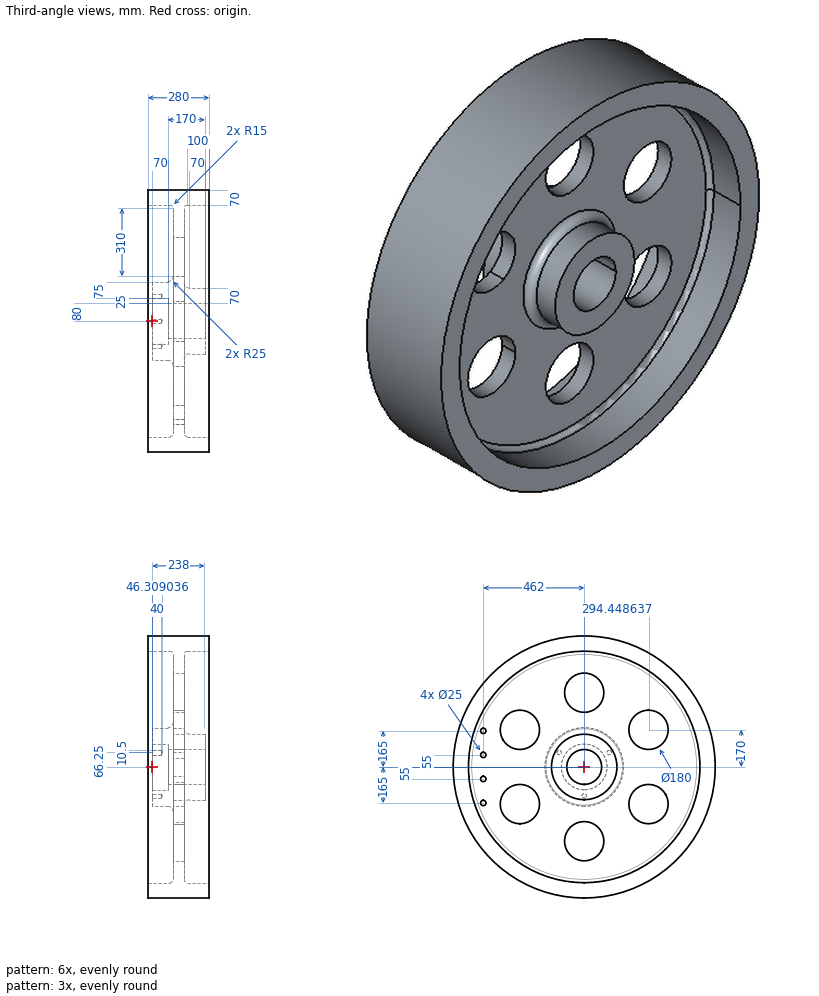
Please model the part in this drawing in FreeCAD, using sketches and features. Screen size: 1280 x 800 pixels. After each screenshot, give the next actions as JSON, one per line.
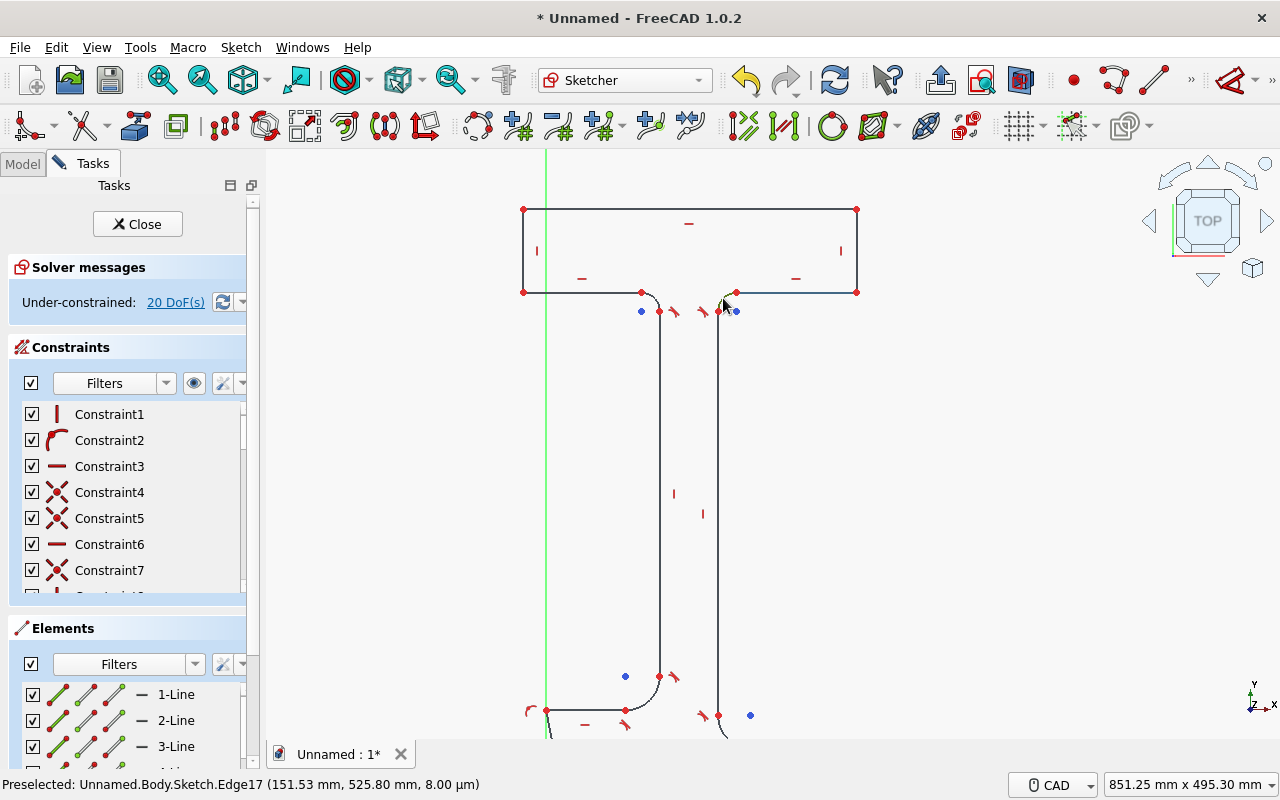
{"action": "key", "text": "t"}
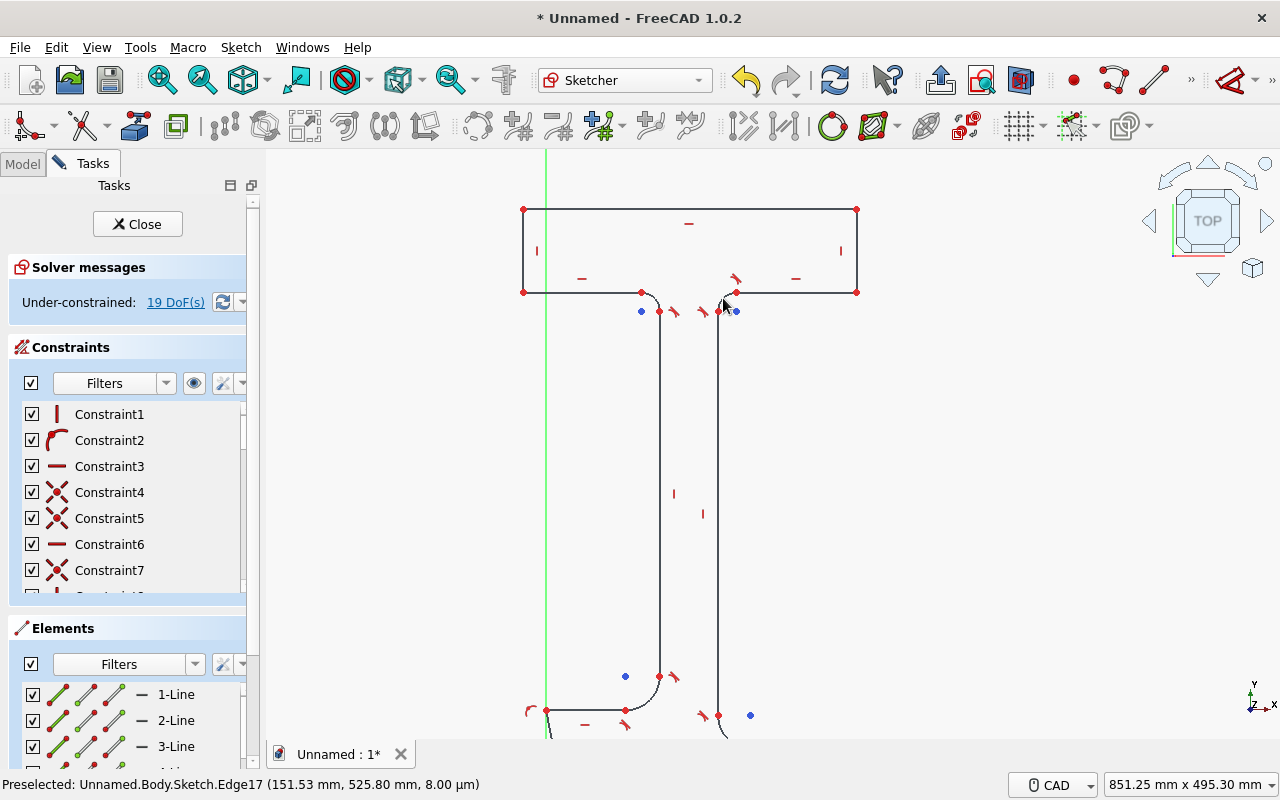
{"action": "left_click", "coordinate": [559, 293]}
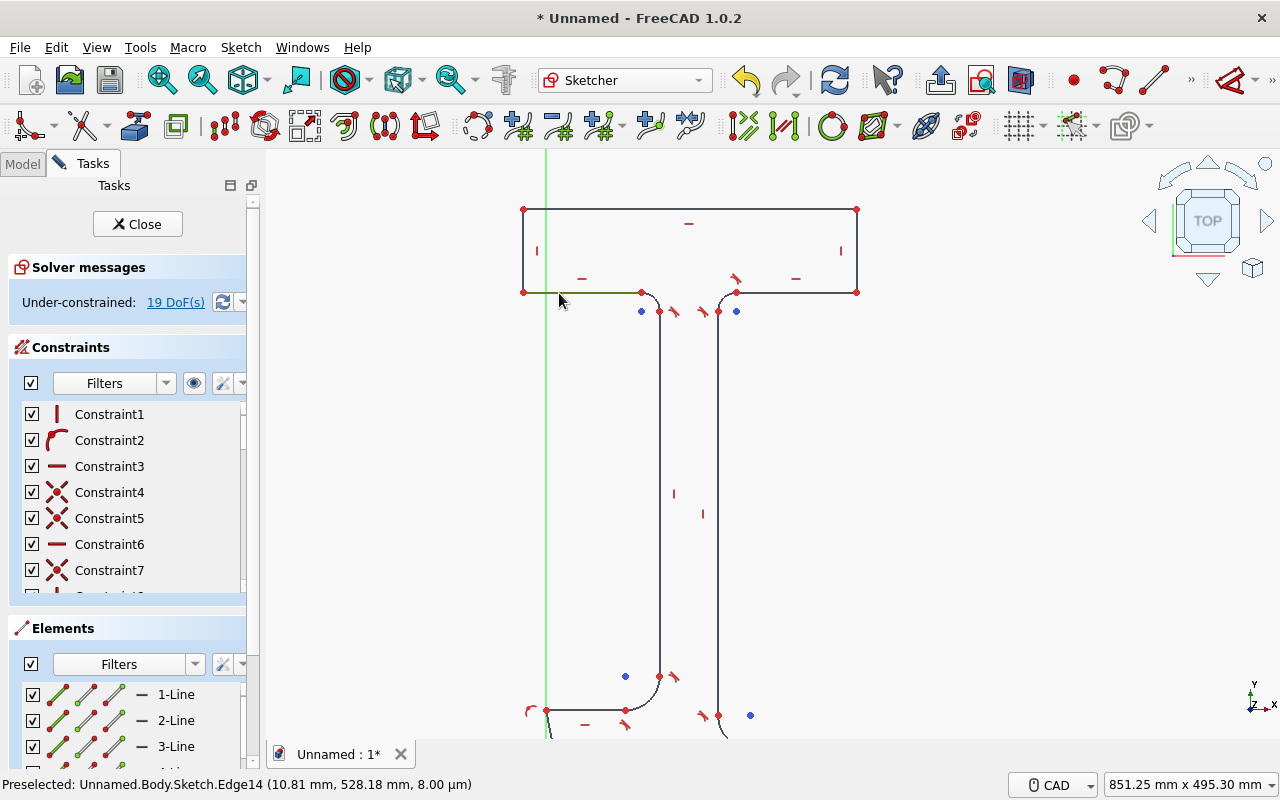
{"action": "left_click", "coordinate": [654, 298]}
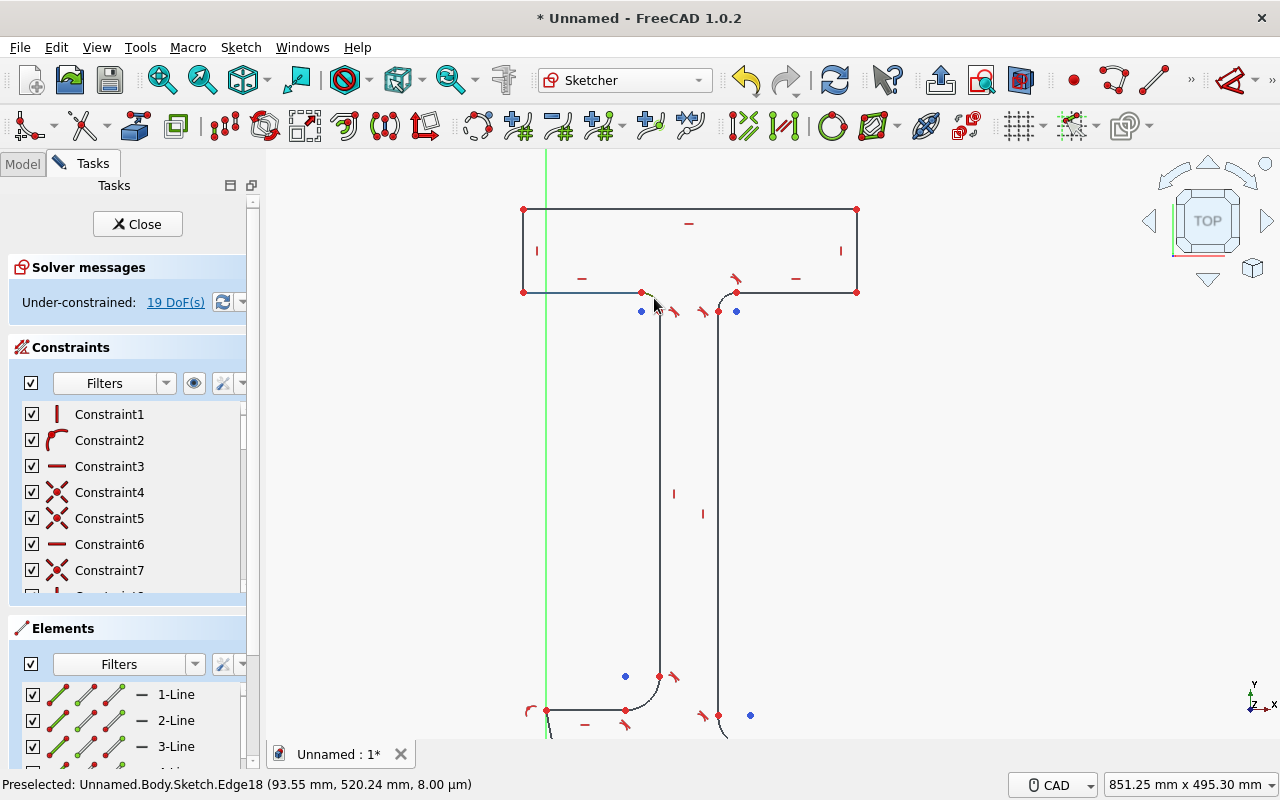
{"action": "key", "text": "t"}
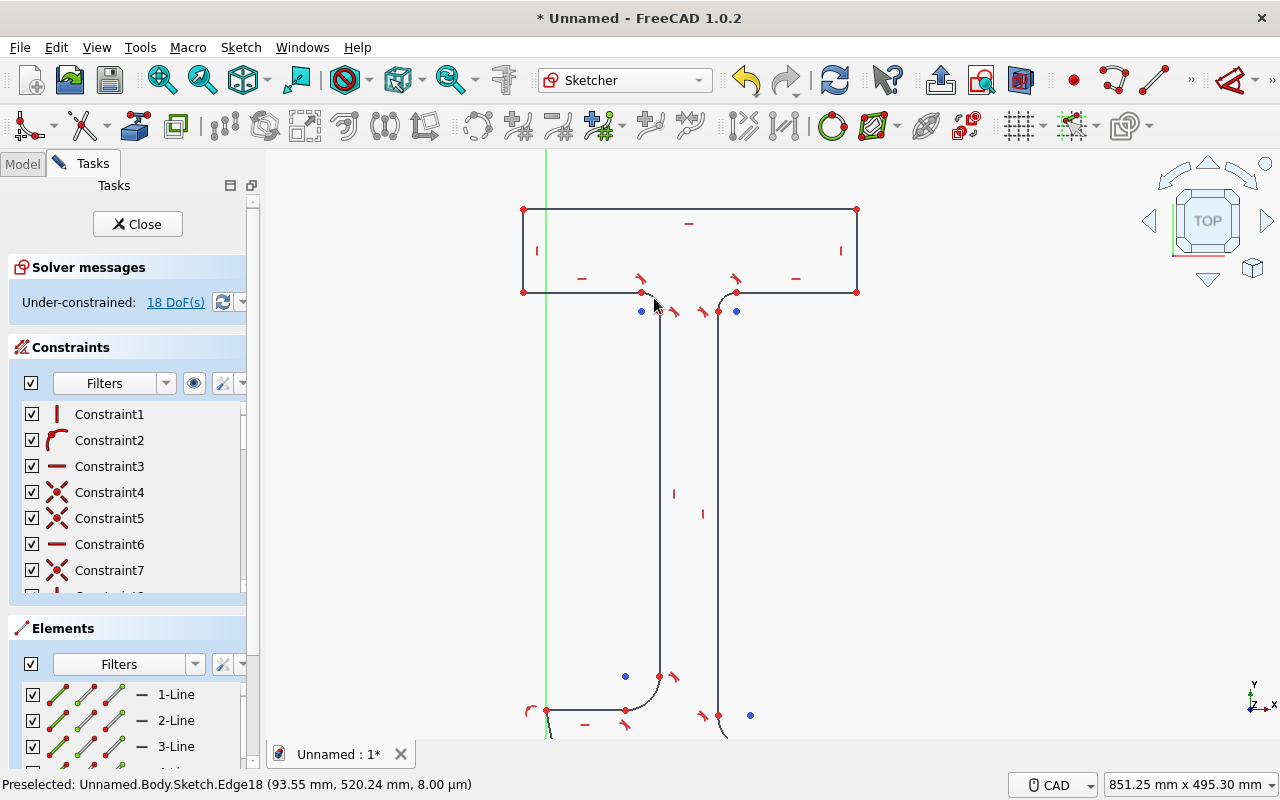
{"action": "scroll", "coordinate": [723, 297], "scroll_direction": "down", "scroll_amount": 3}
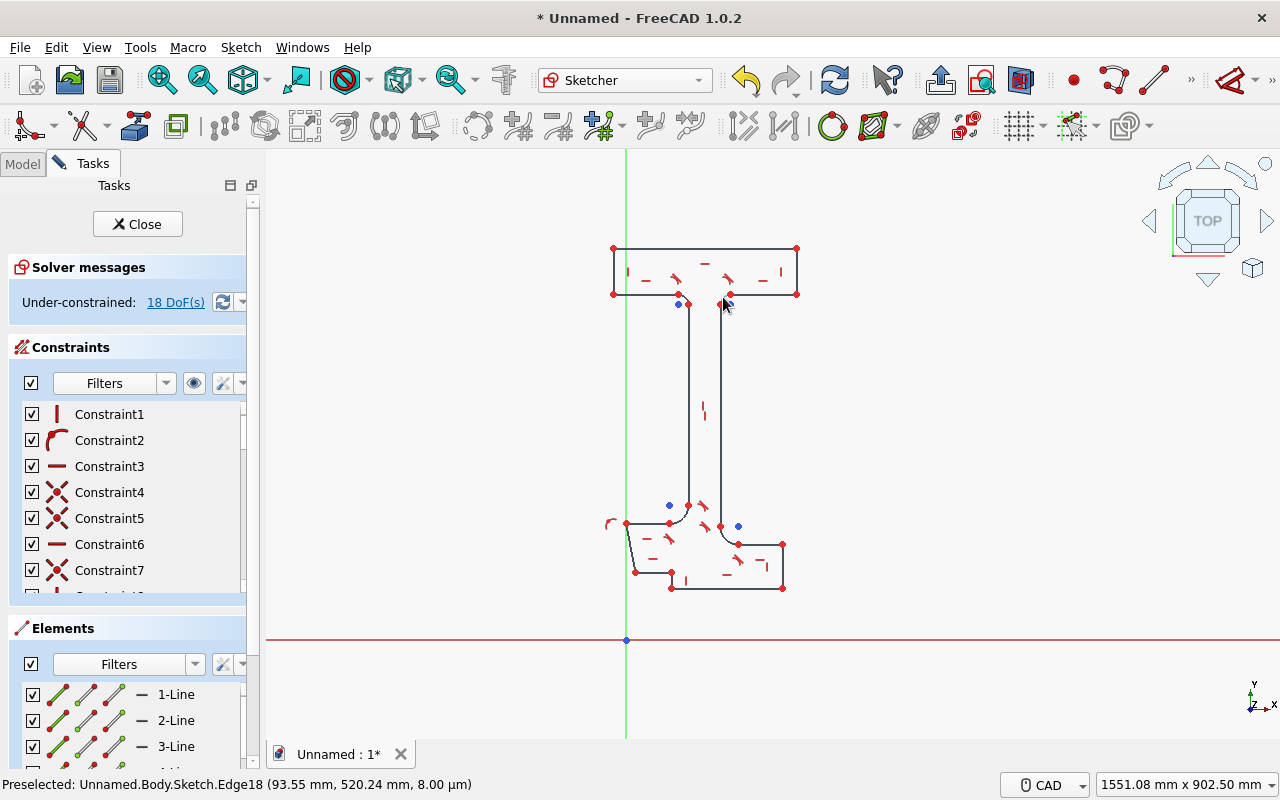
{"action": "scroll", "coordinate": [633, 558], "scroll_direction": "up", "scroll_amount": 4}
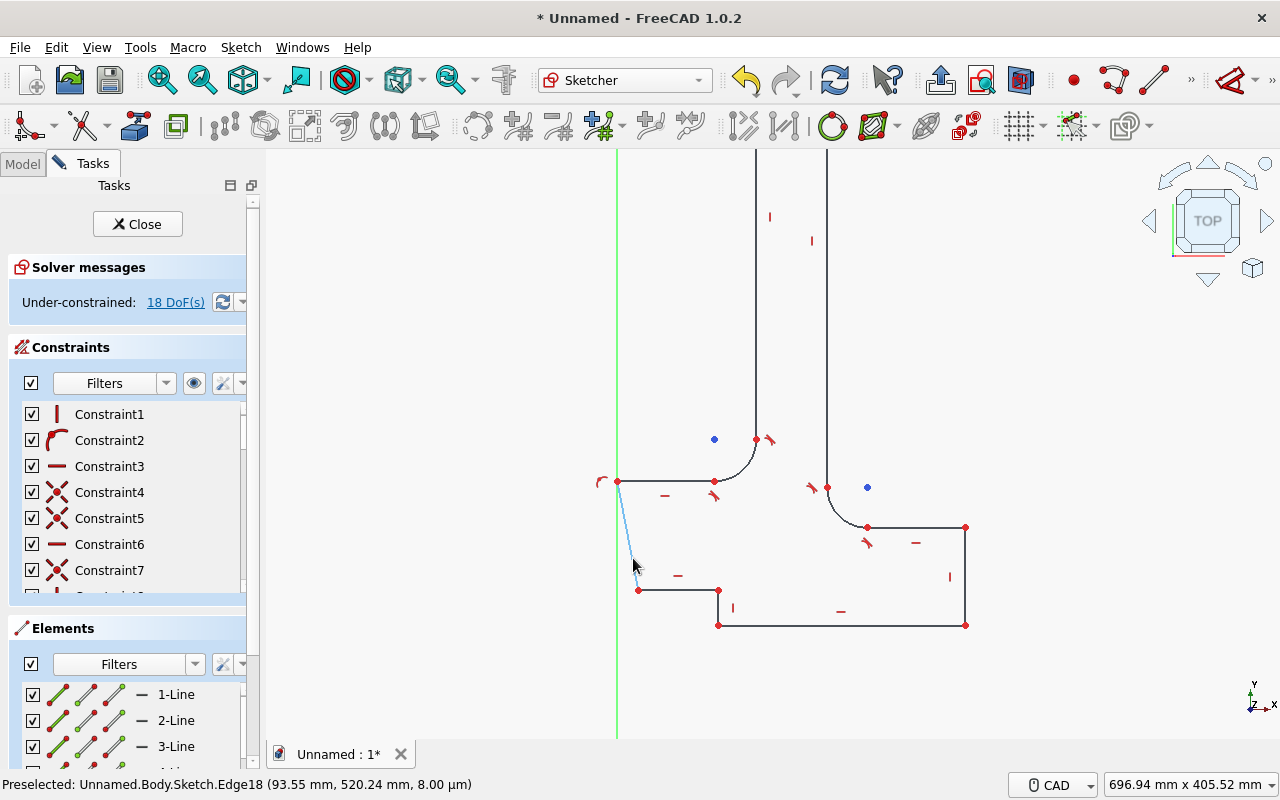
{"action": "left_click", "coordinate": [632, 558]}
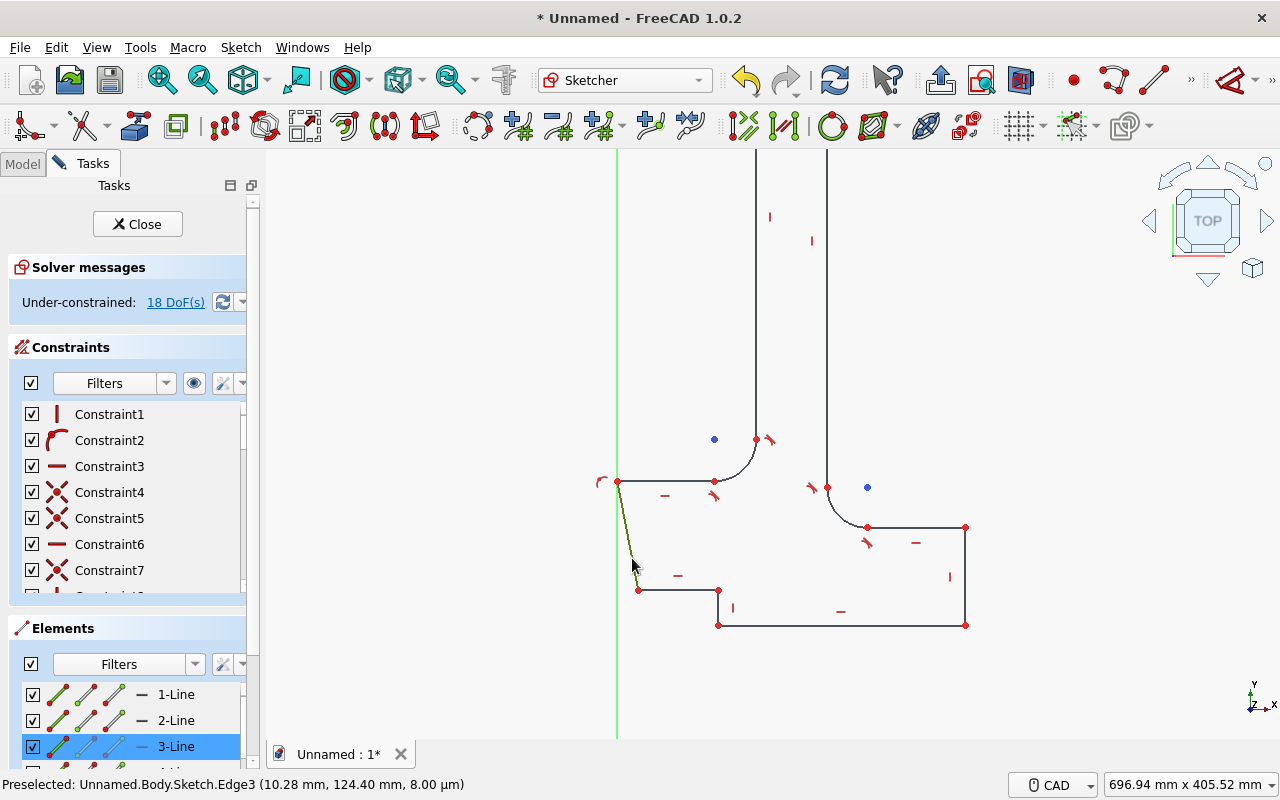
{"action": "key", "text": "v"}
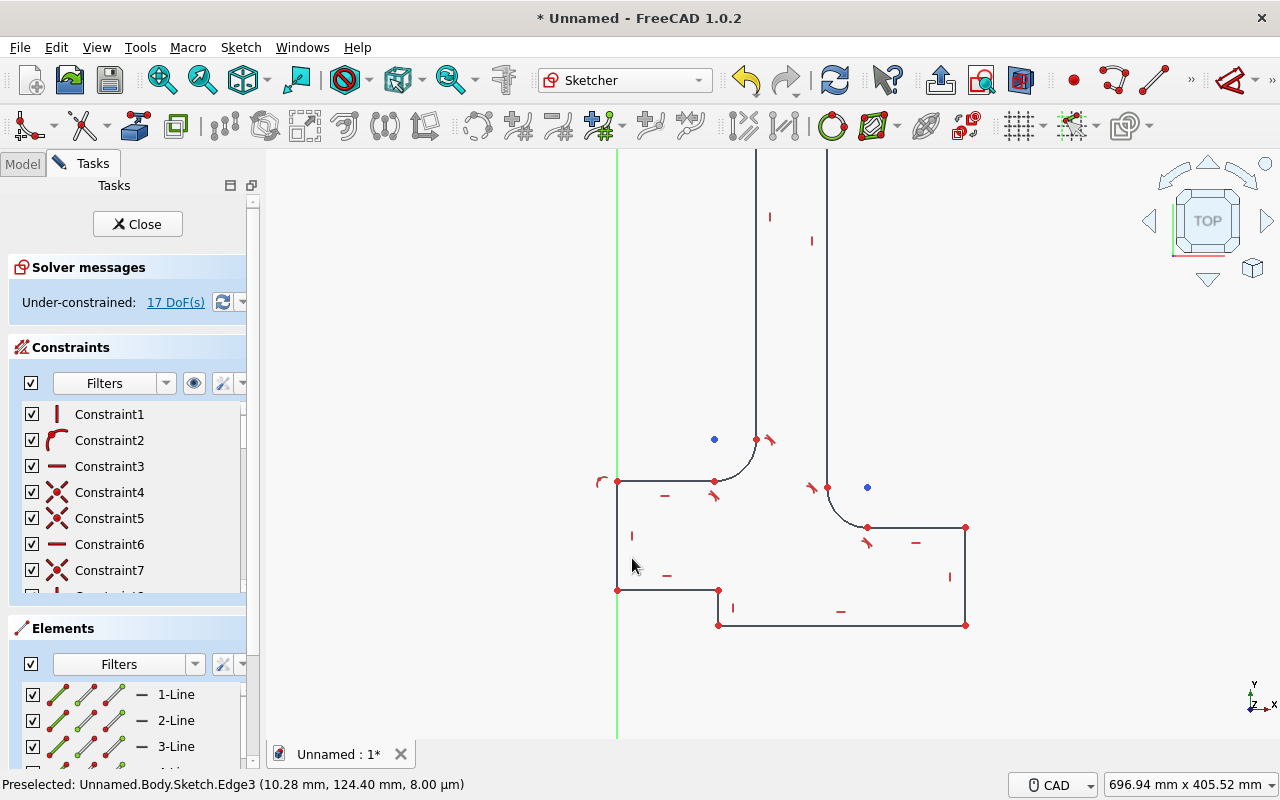
{"action": "left_click", "coordinate": [733, 477]}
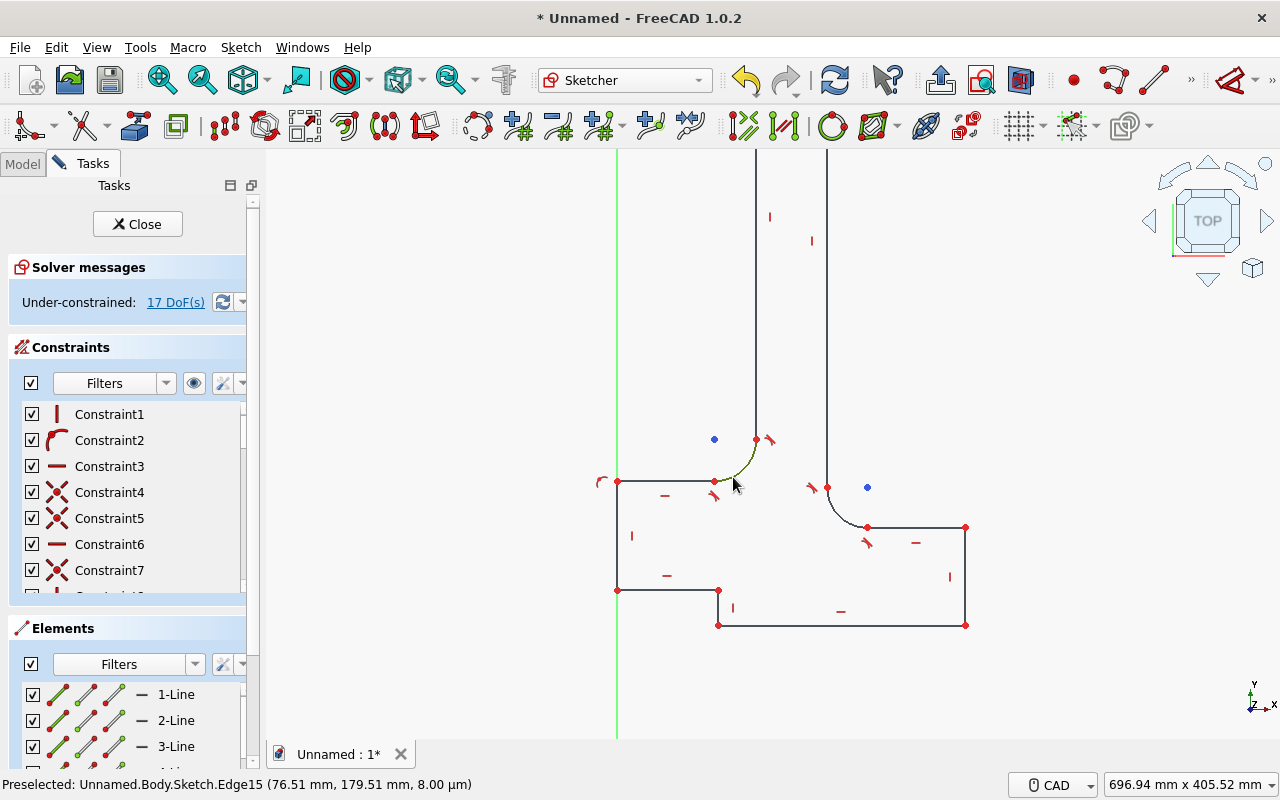
{"action": "left_click", "coordinate": [832, 506]}